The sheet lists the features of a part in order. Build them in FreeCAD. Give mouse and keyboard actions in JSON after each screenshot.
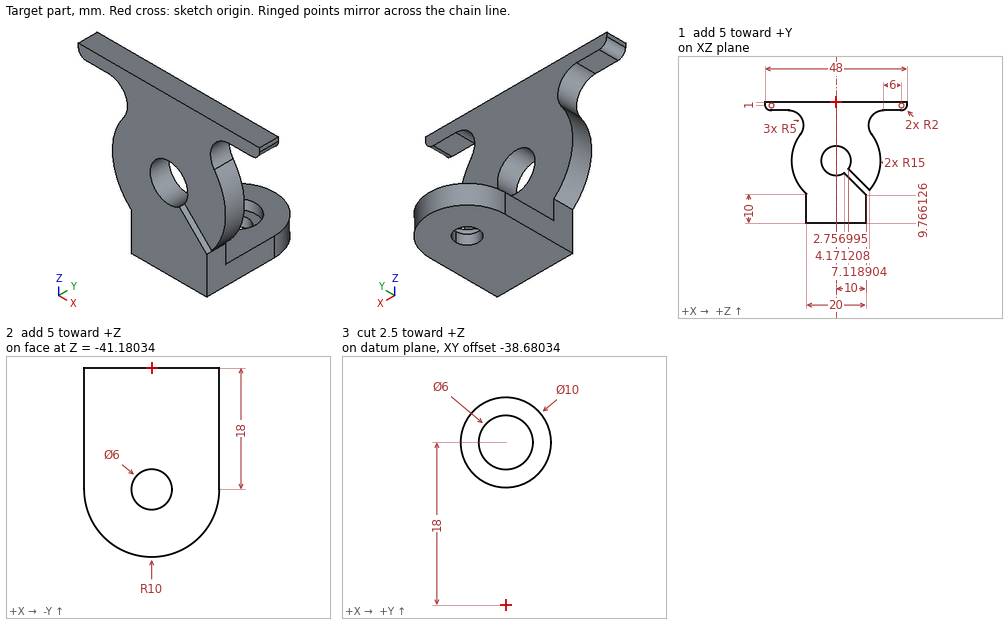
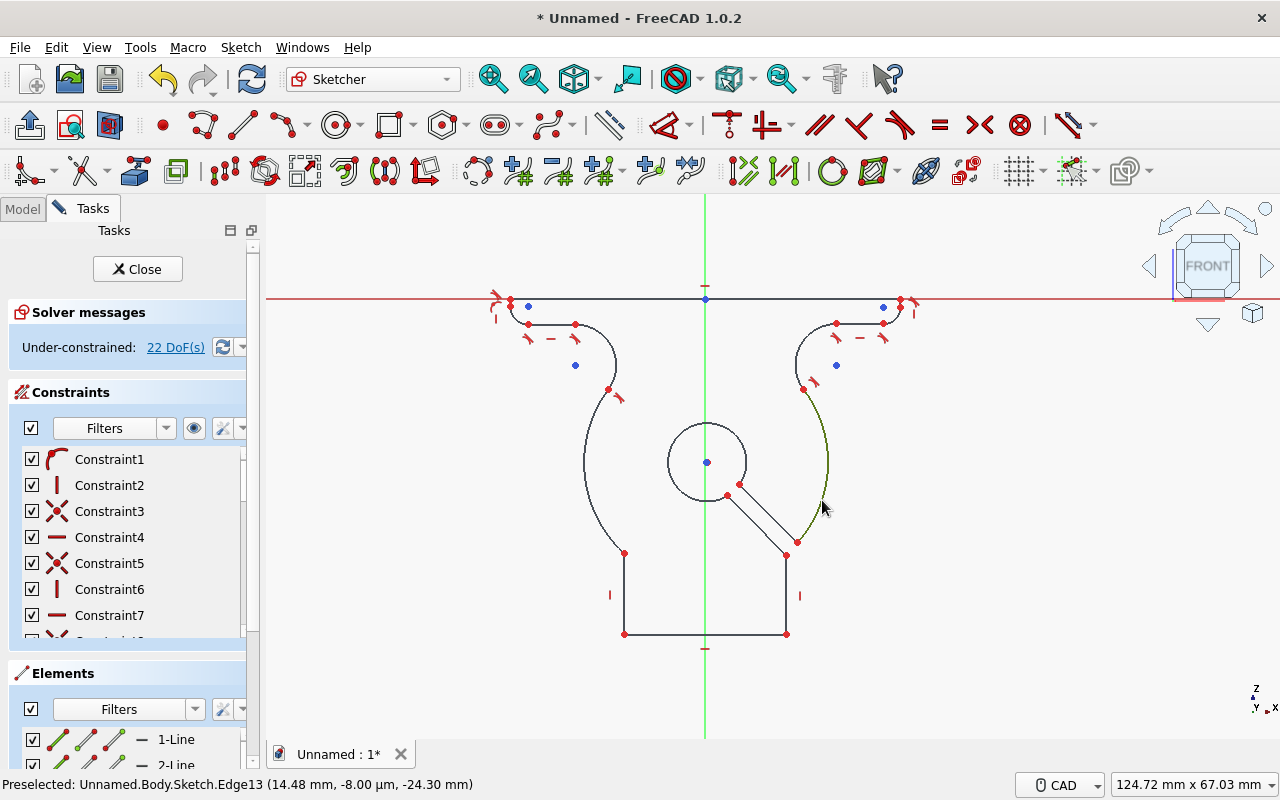
{"action": "left_click", "coordinate": [586, 439]}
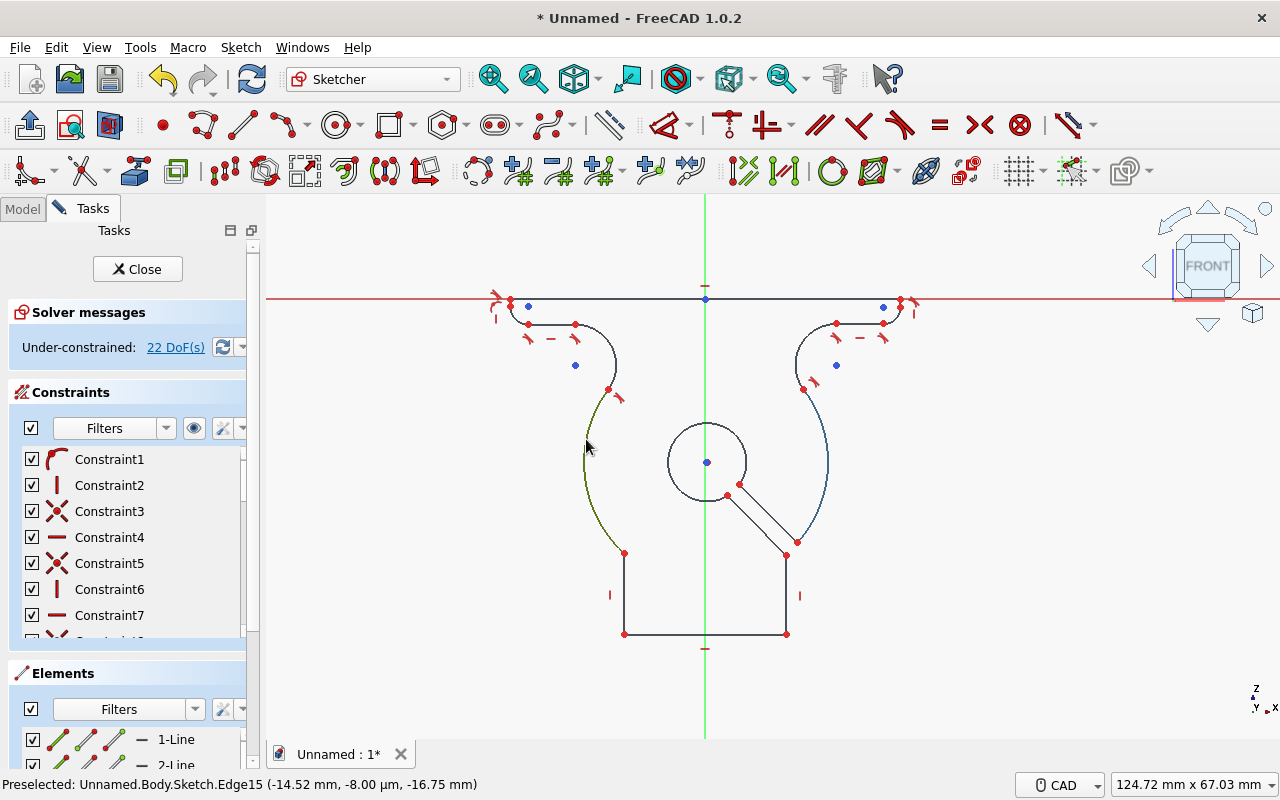
{"action": "key", "text": "c"}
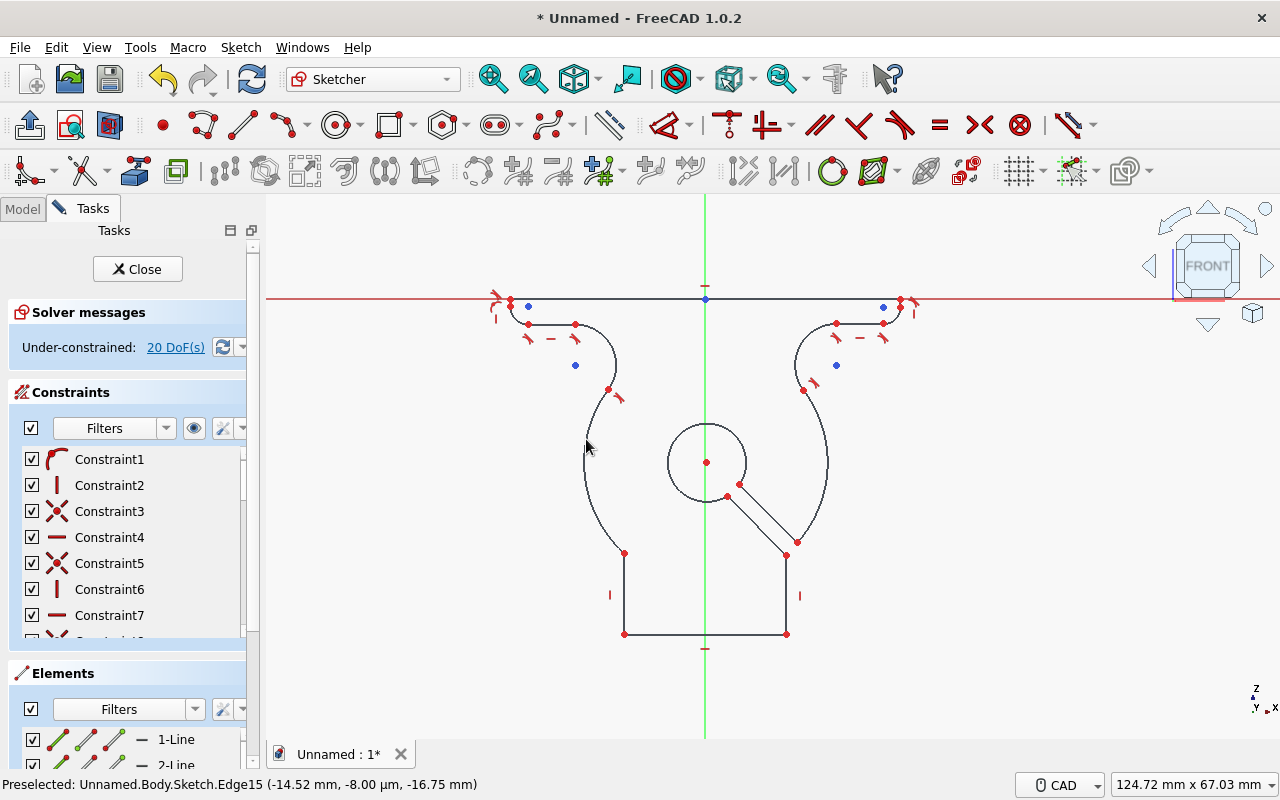
{"action": "left_click", "coordinate": [811, 333]}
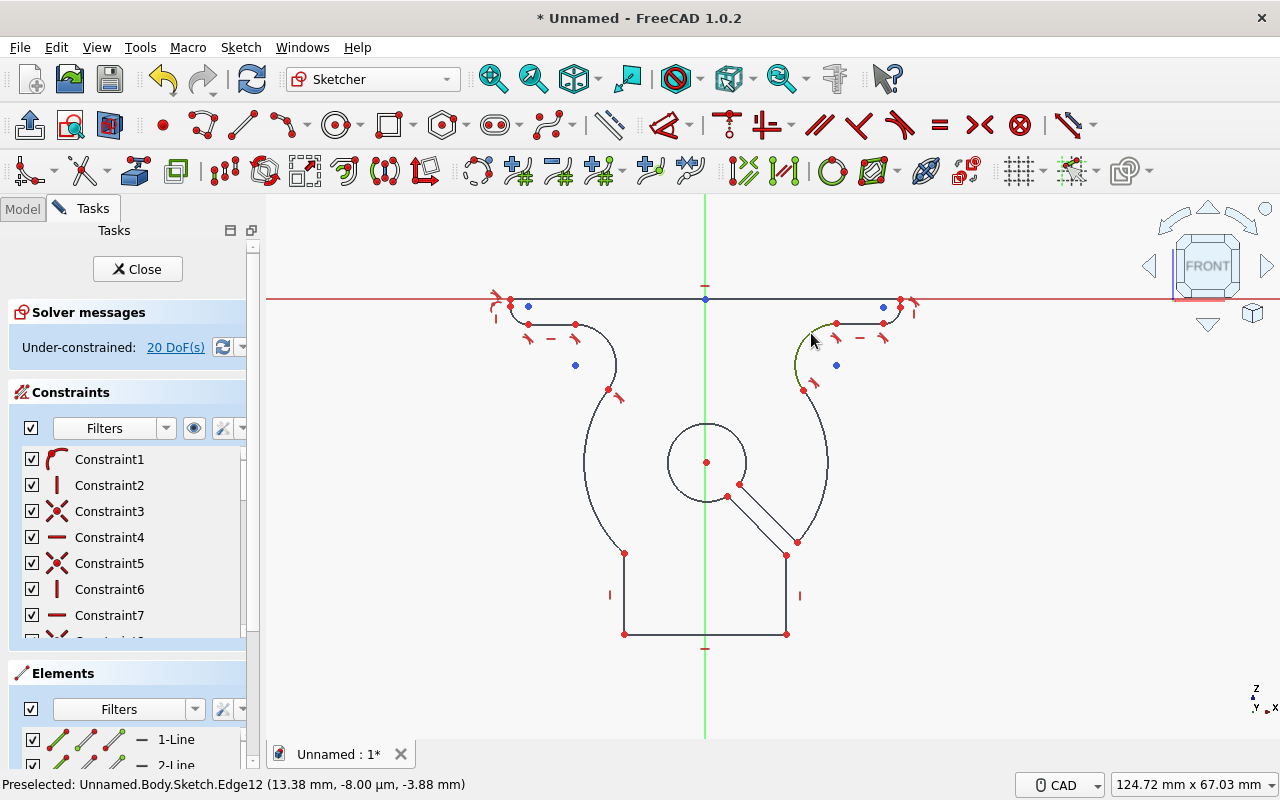
{"action": "left_click", "coordinate": [723, 427]}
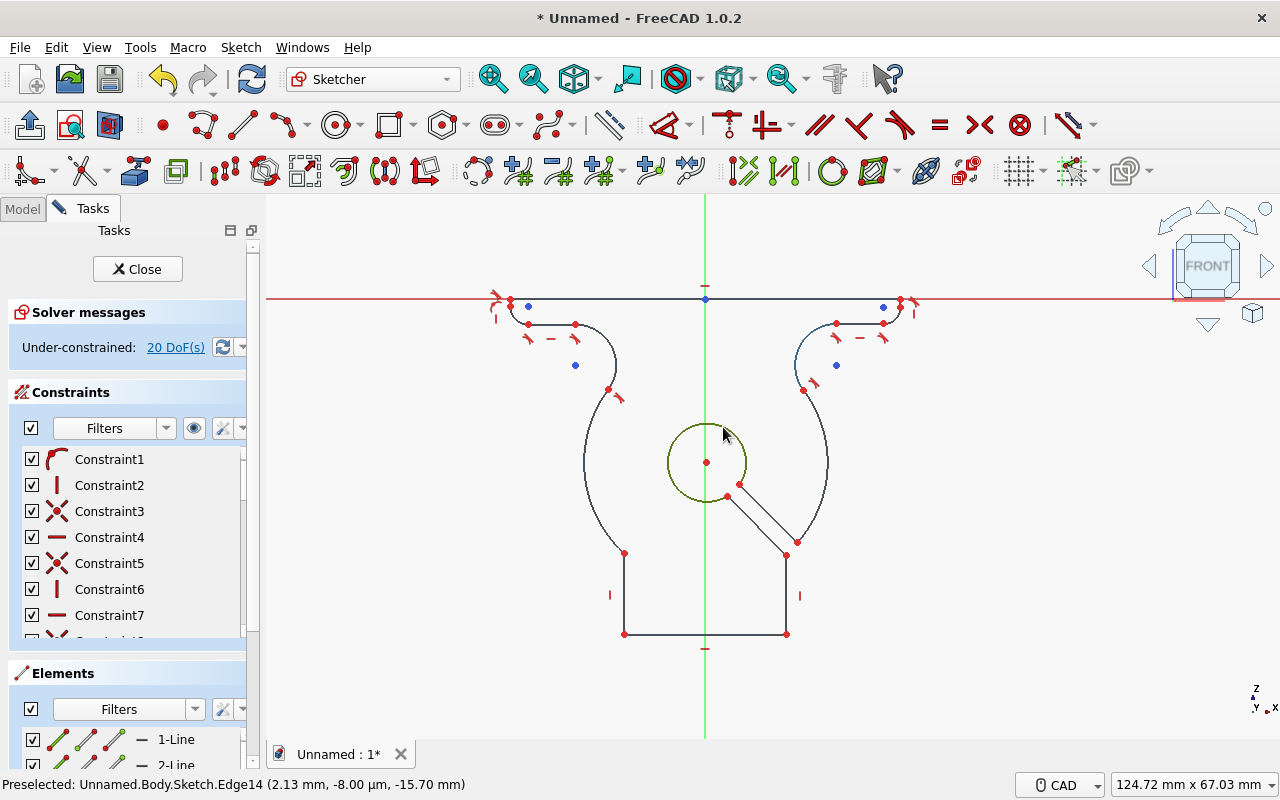
{"action": "left_click", "coordinate": [616, 364]}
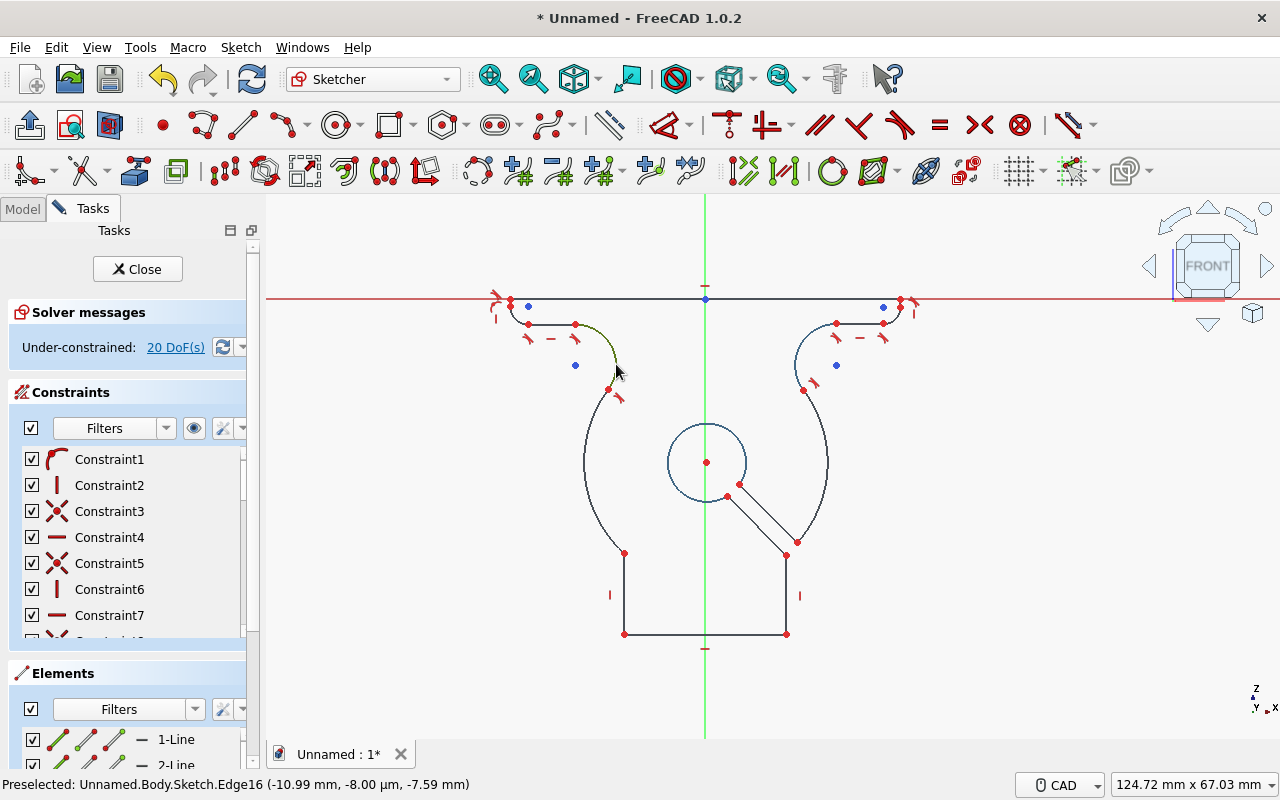
{"action": "key", "text": "e"}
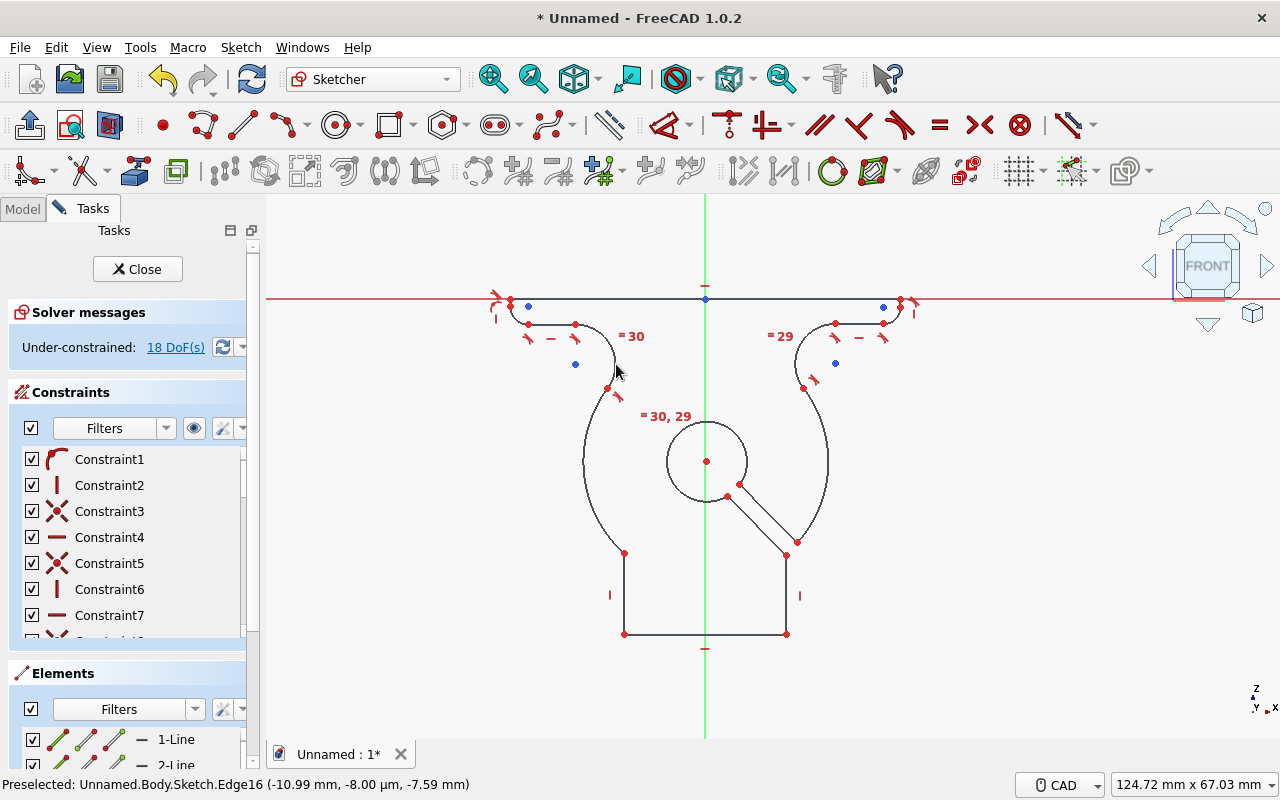
{"action": "left_click", "coordinate": [822, 499]}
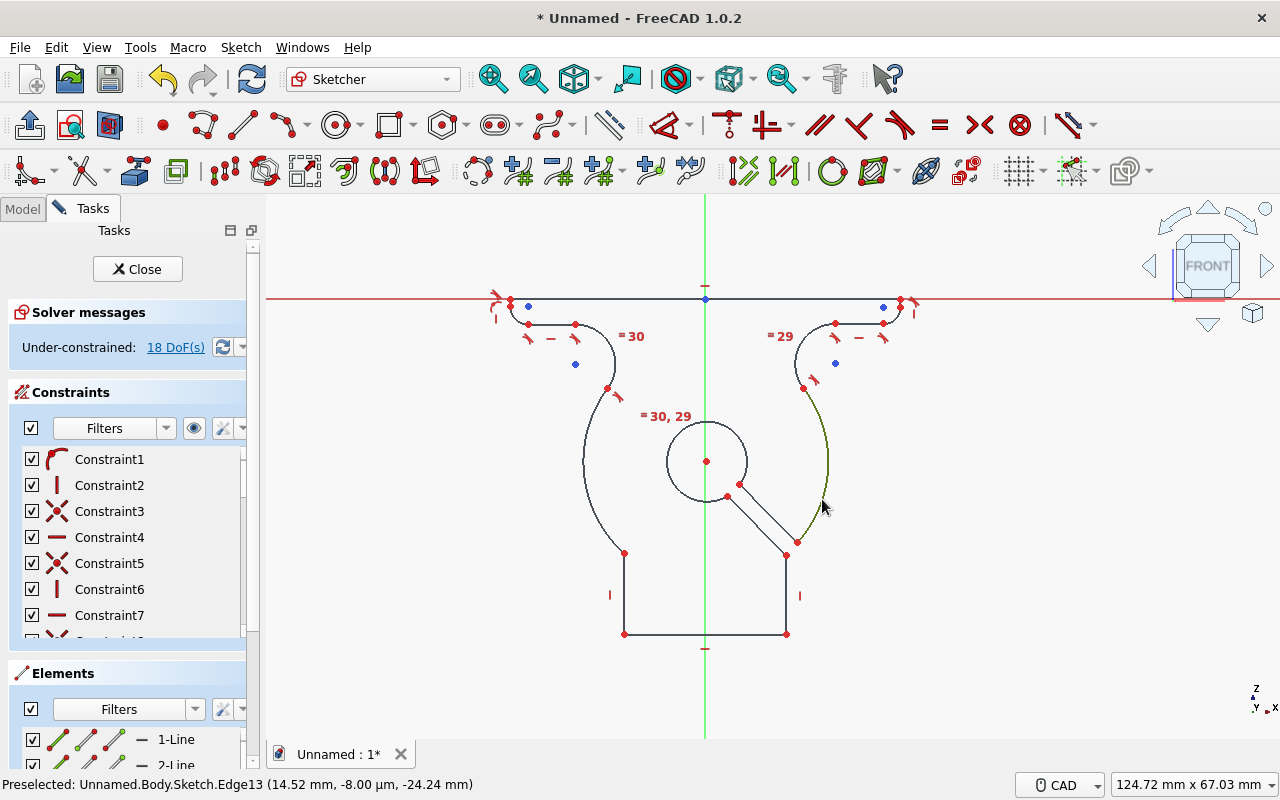
{"action": "left_click", "coordinate": [586, 438]}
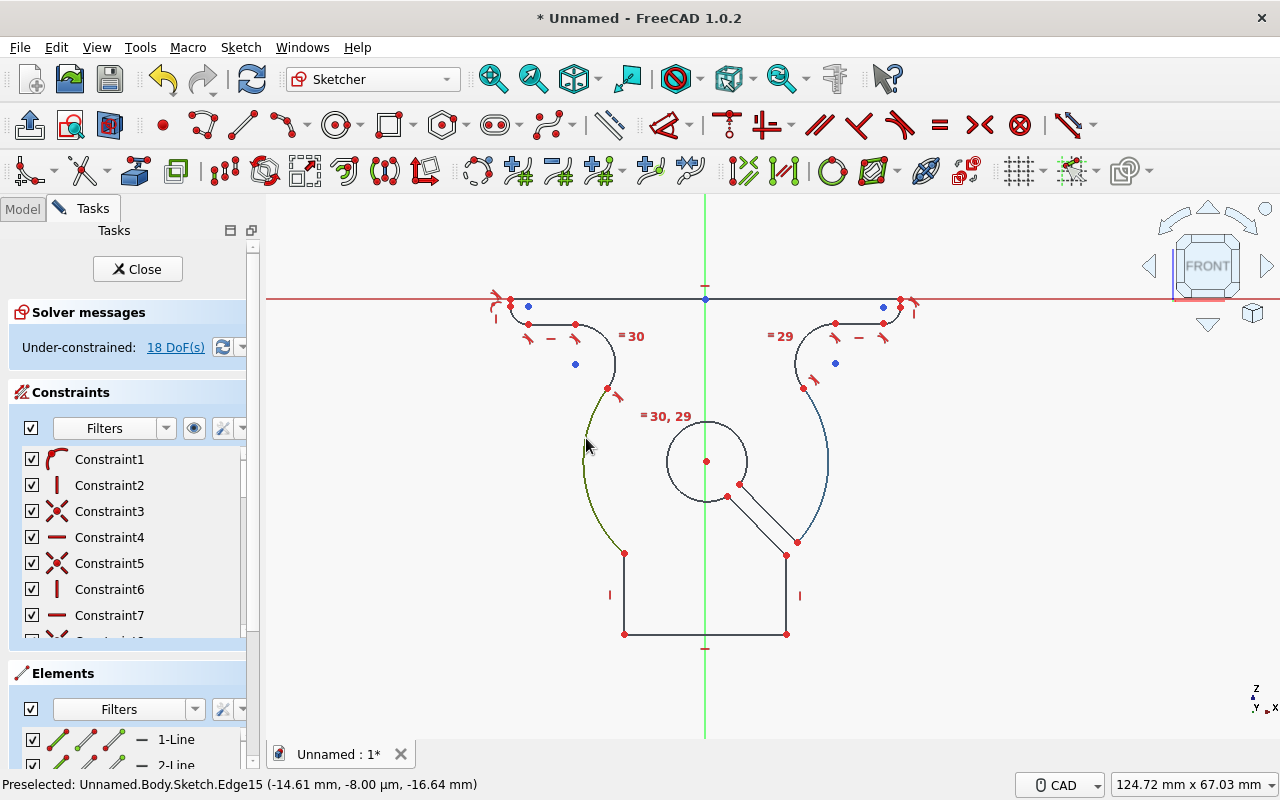
{"action": "key", "text": "e"}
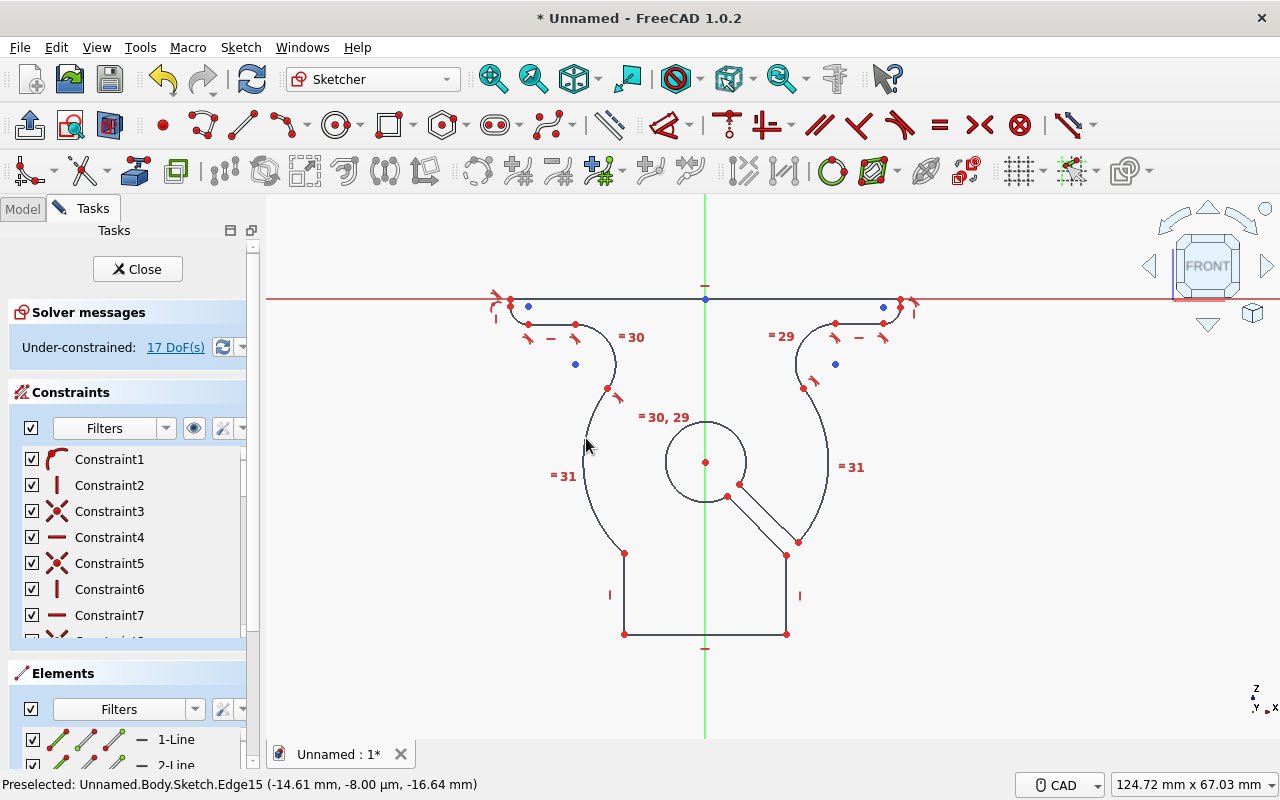
{"action": "left_click", "coordinate": [896, 319]}